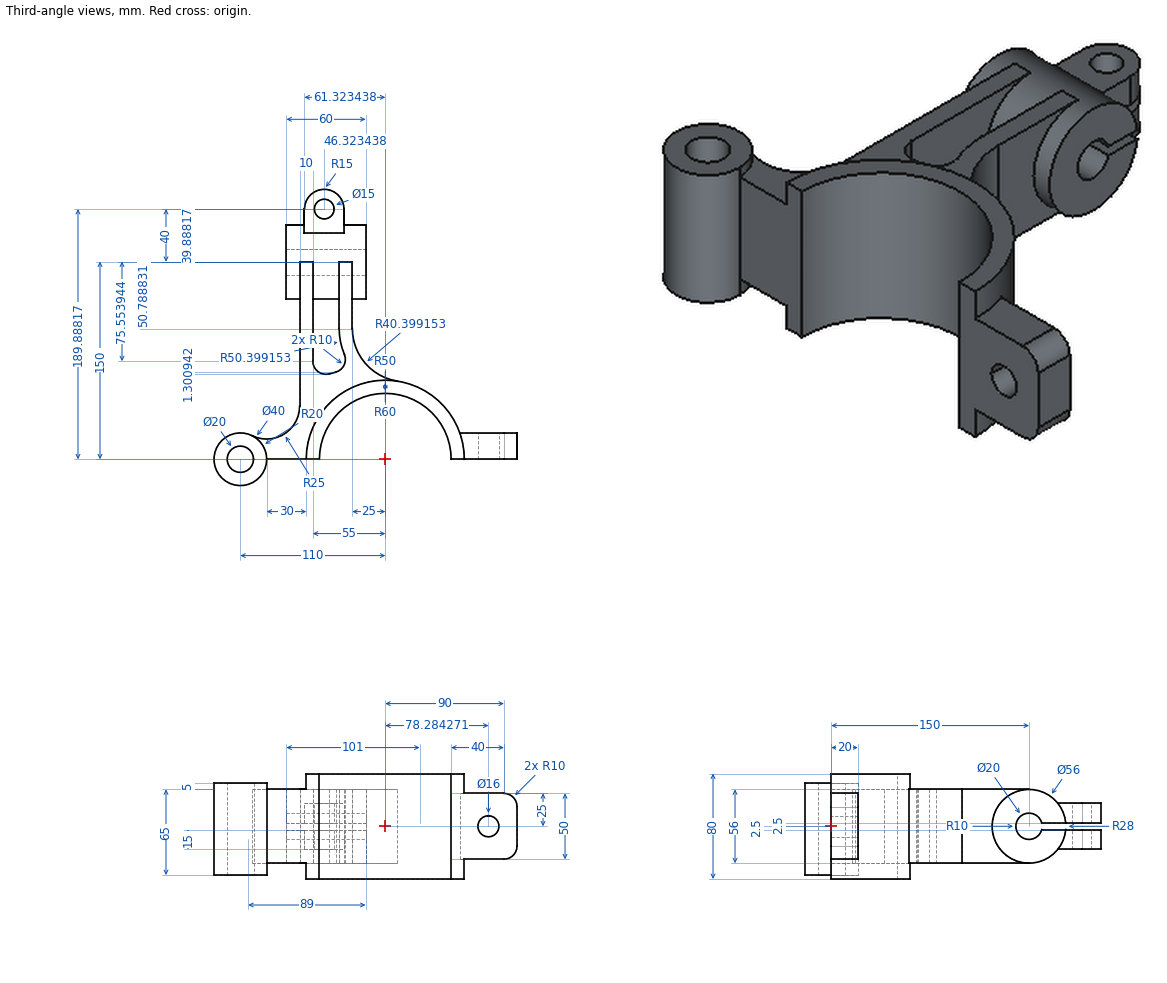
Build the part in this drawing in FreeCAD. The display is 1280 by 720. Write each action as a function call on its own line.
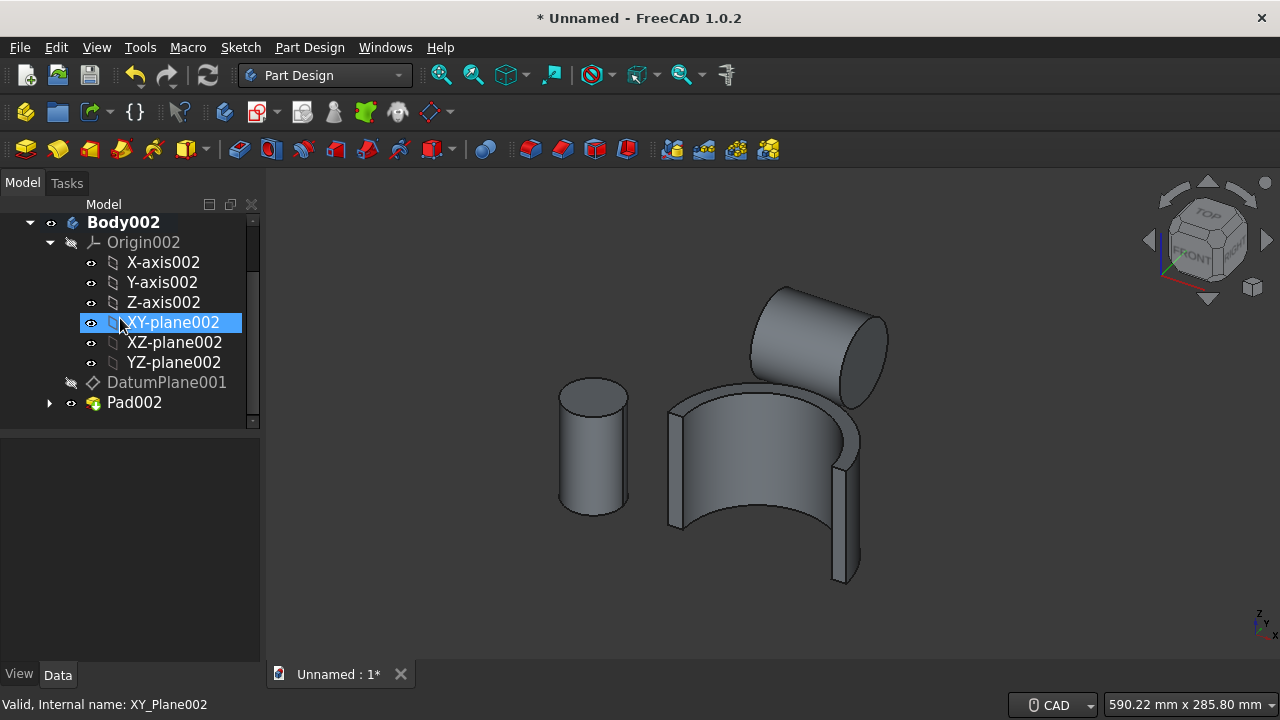
scroll(120, 318, up, 15)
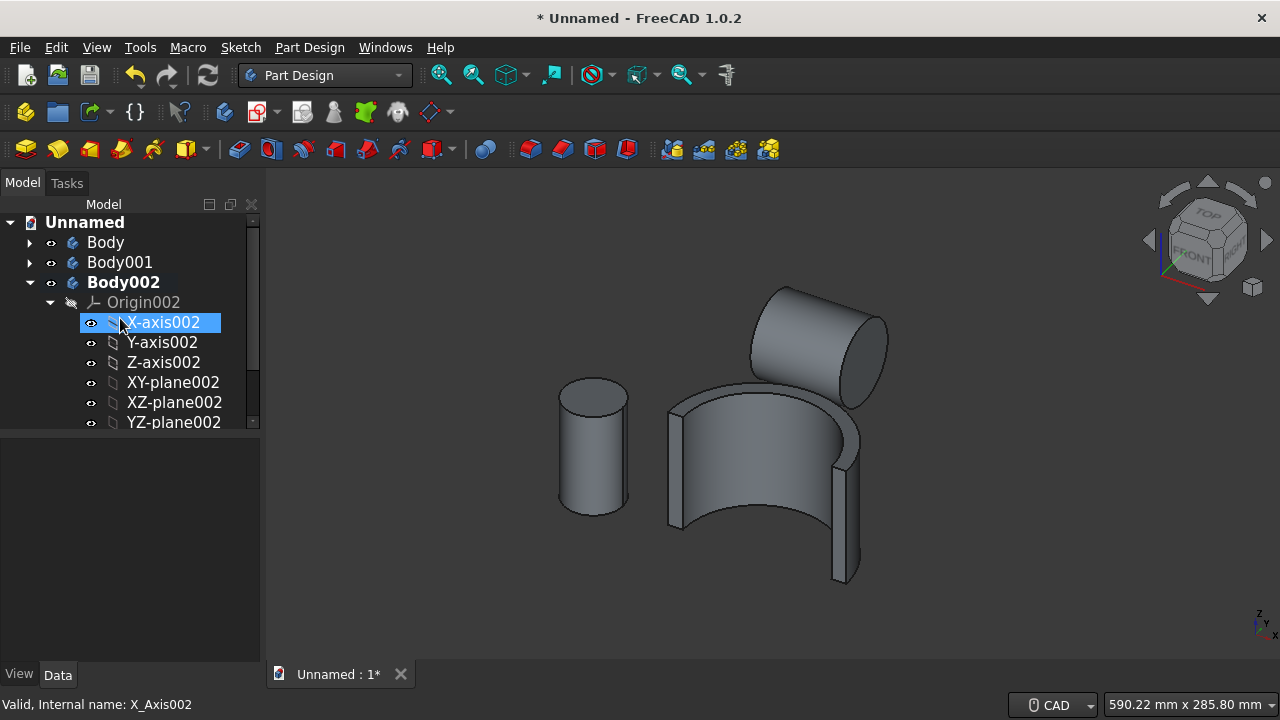
double_click(96, 243)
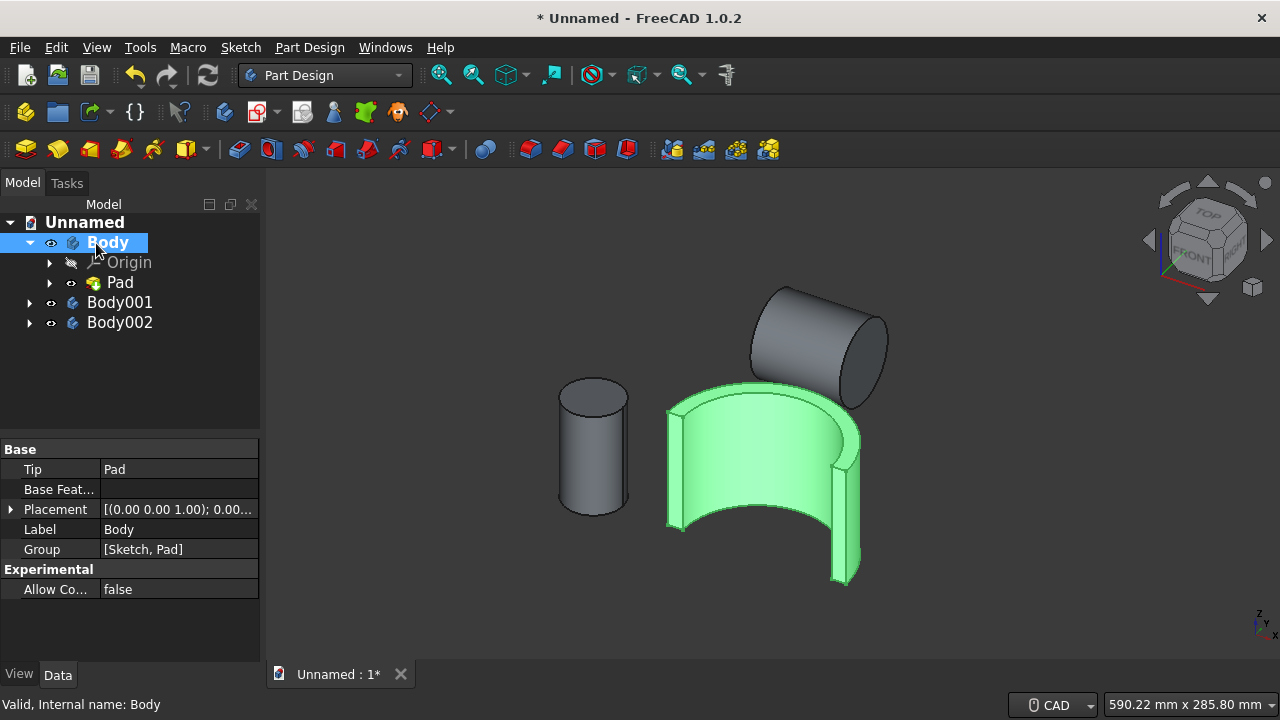
click(96, 243)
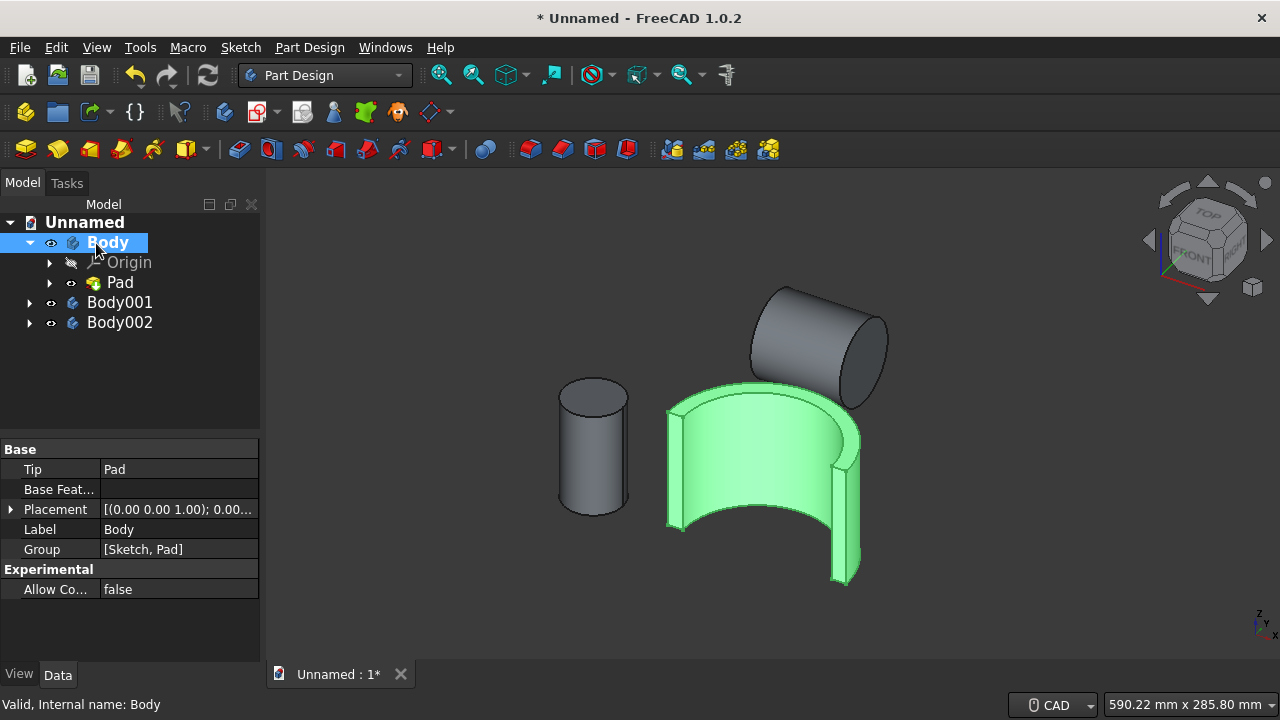
click(146, 589)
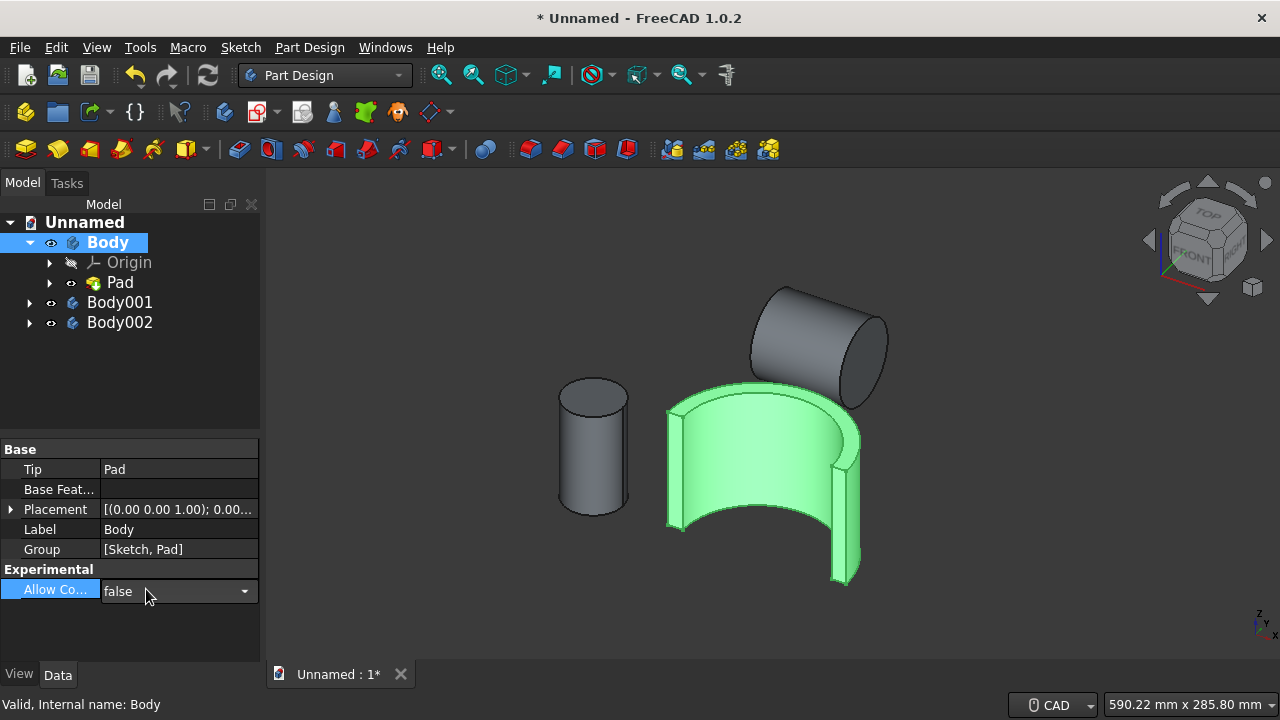
click(146, 589)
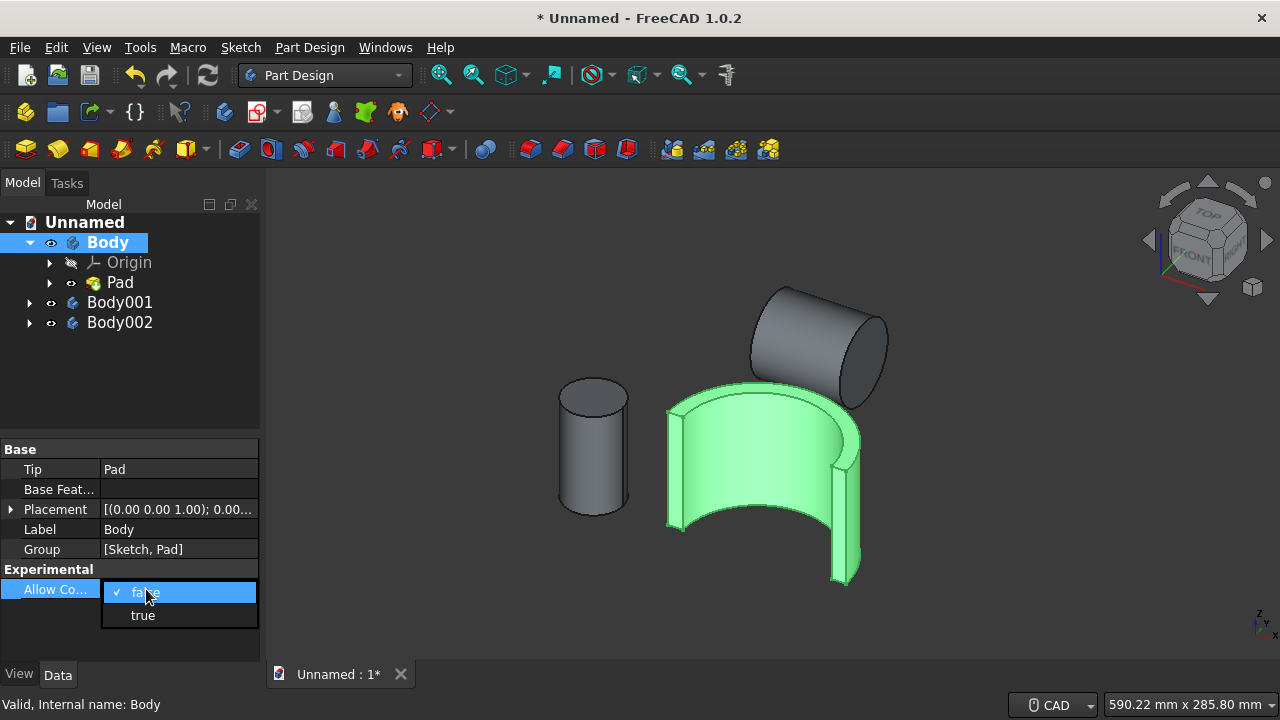
click(179, 616)
key(Return)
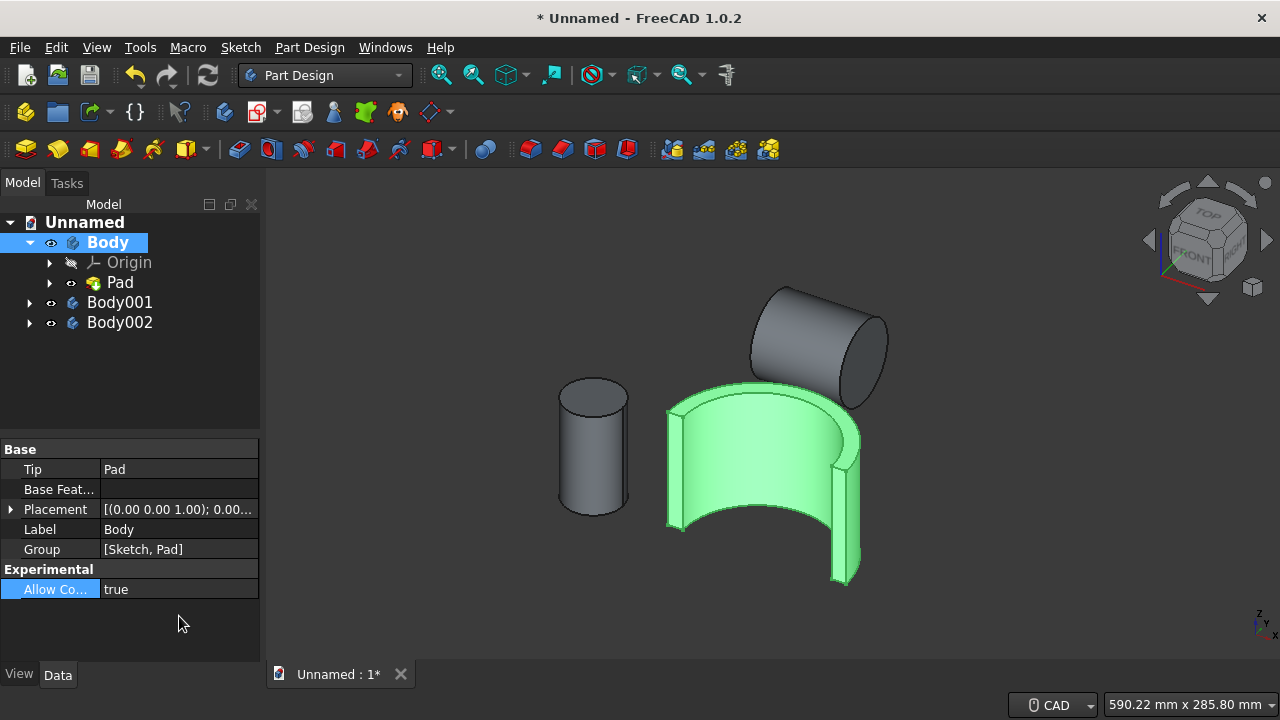
click(96, 303)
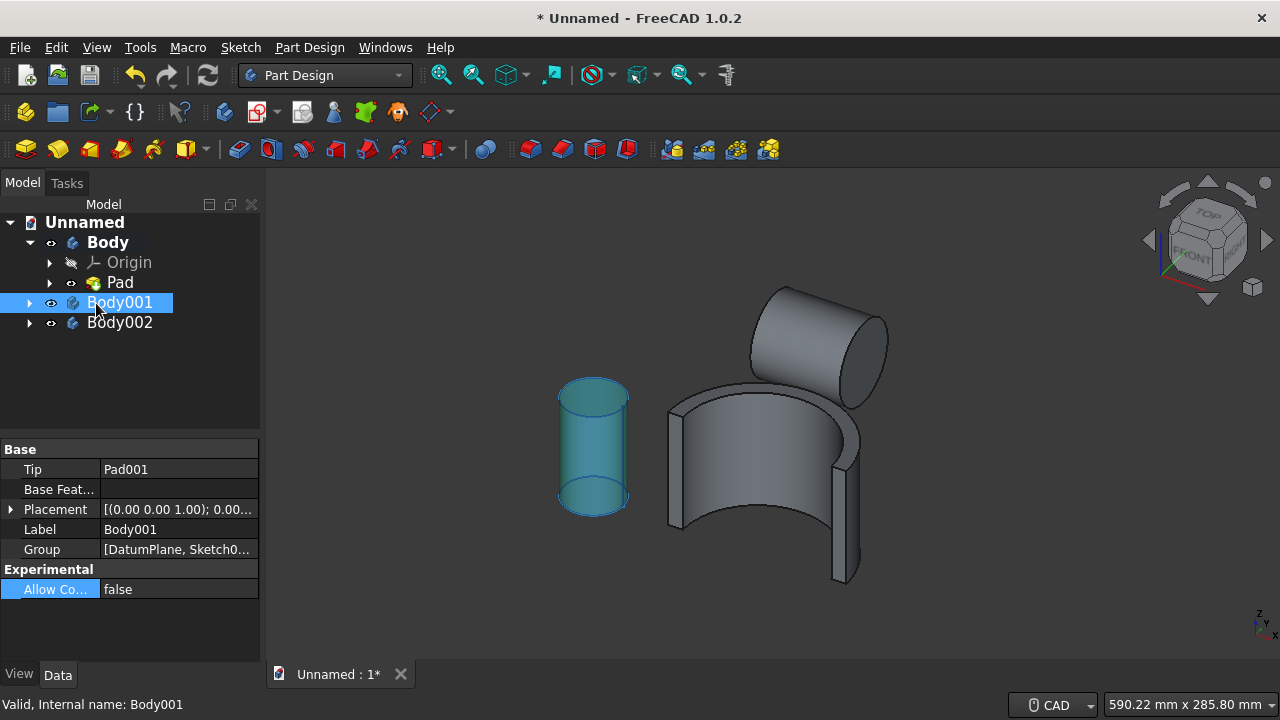
click(486, 150)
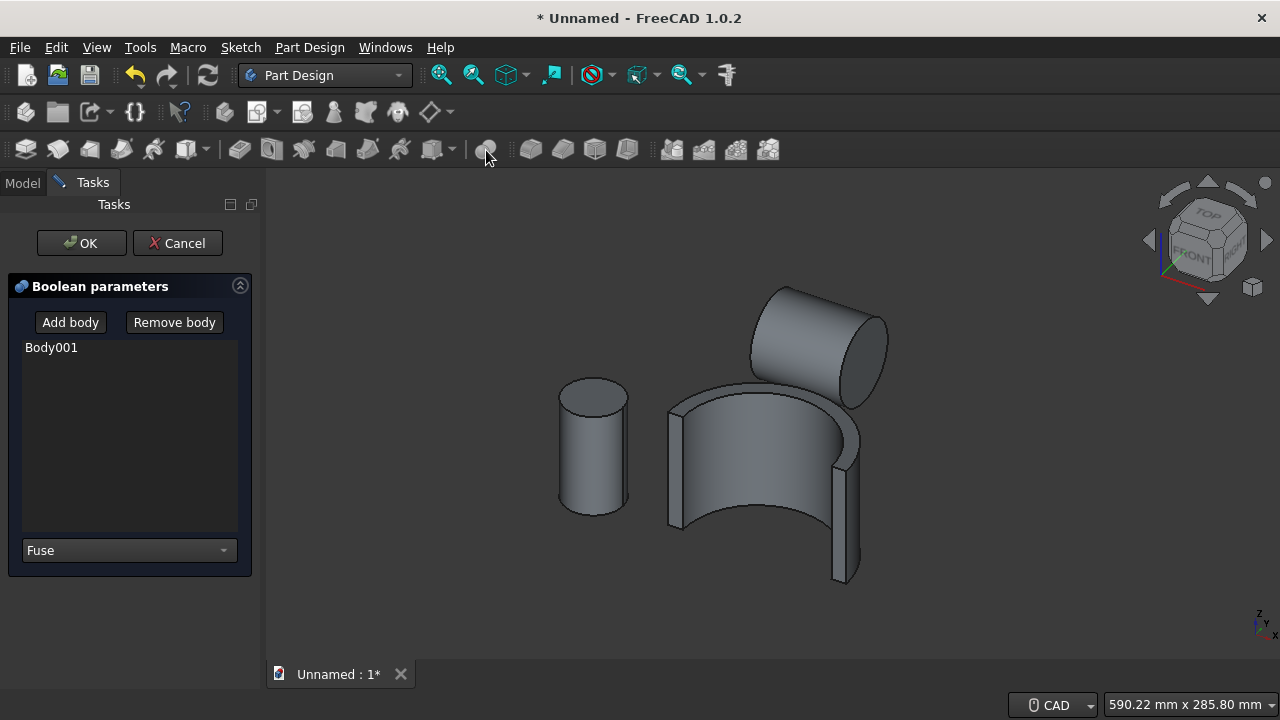
click(82, 243)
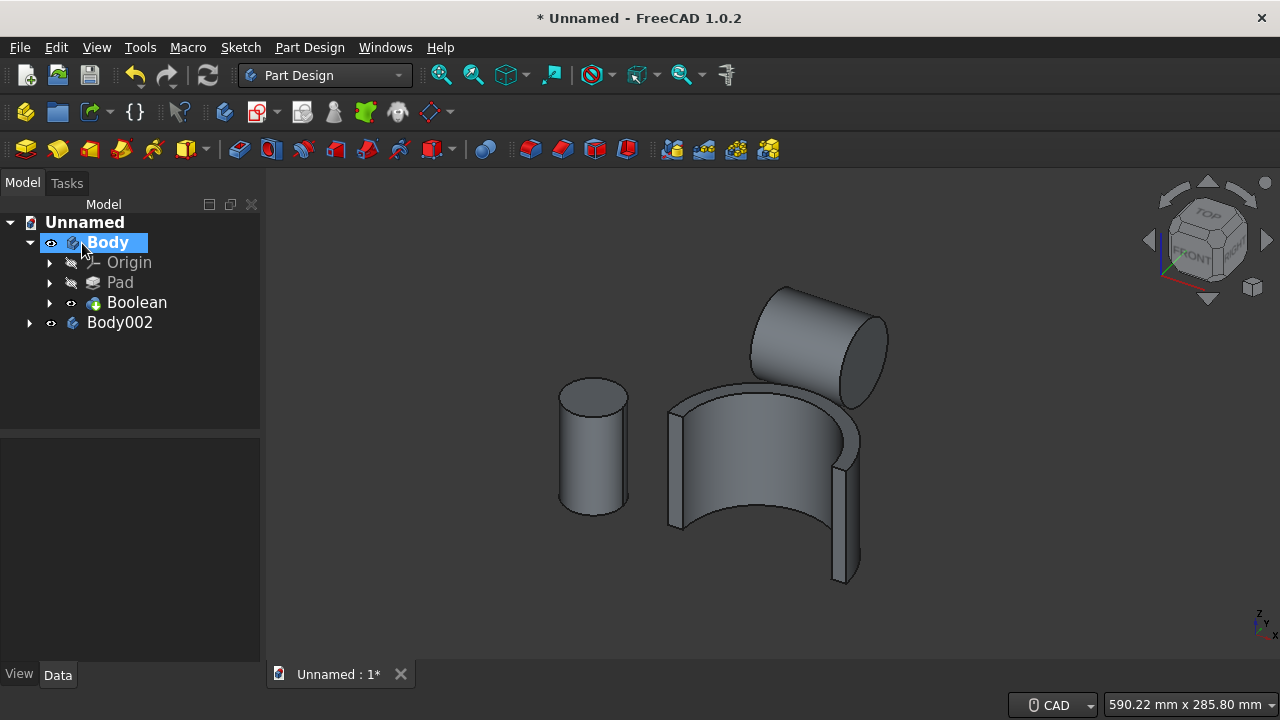
click(96, 323)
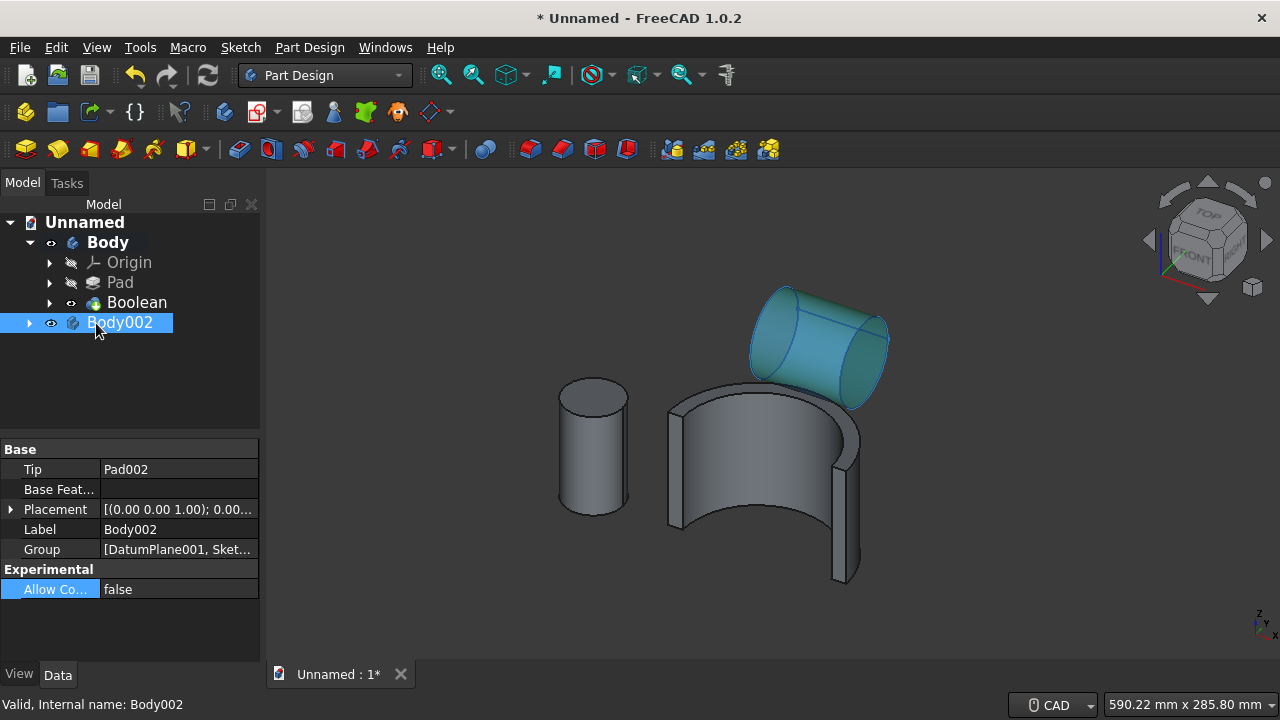
click(486, 150)